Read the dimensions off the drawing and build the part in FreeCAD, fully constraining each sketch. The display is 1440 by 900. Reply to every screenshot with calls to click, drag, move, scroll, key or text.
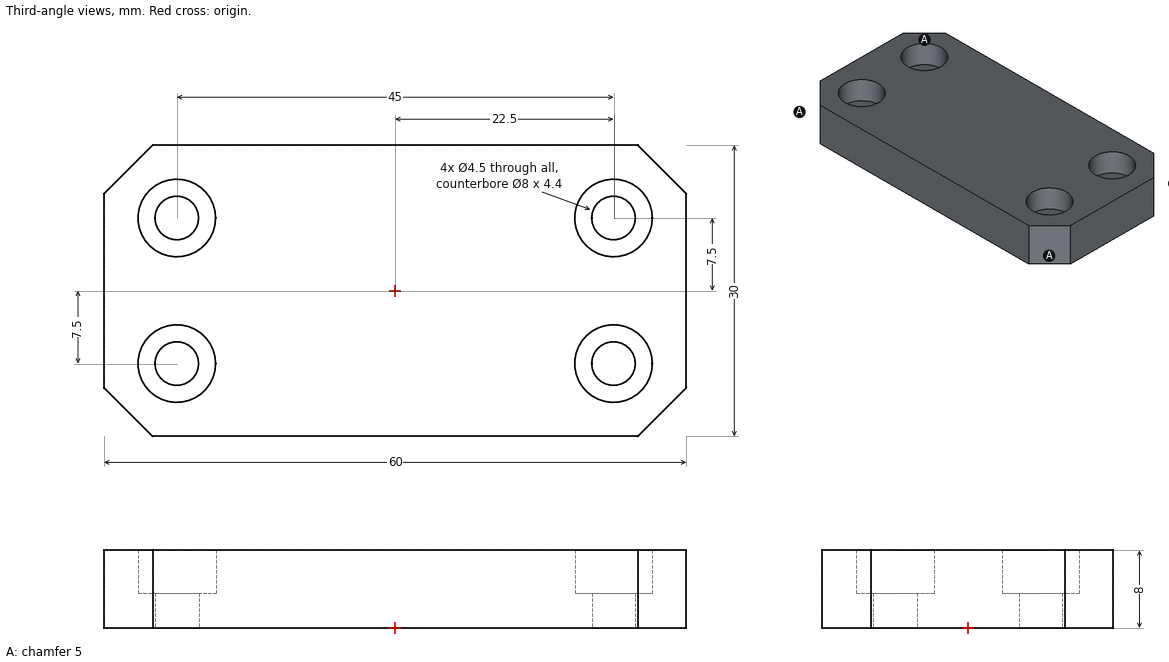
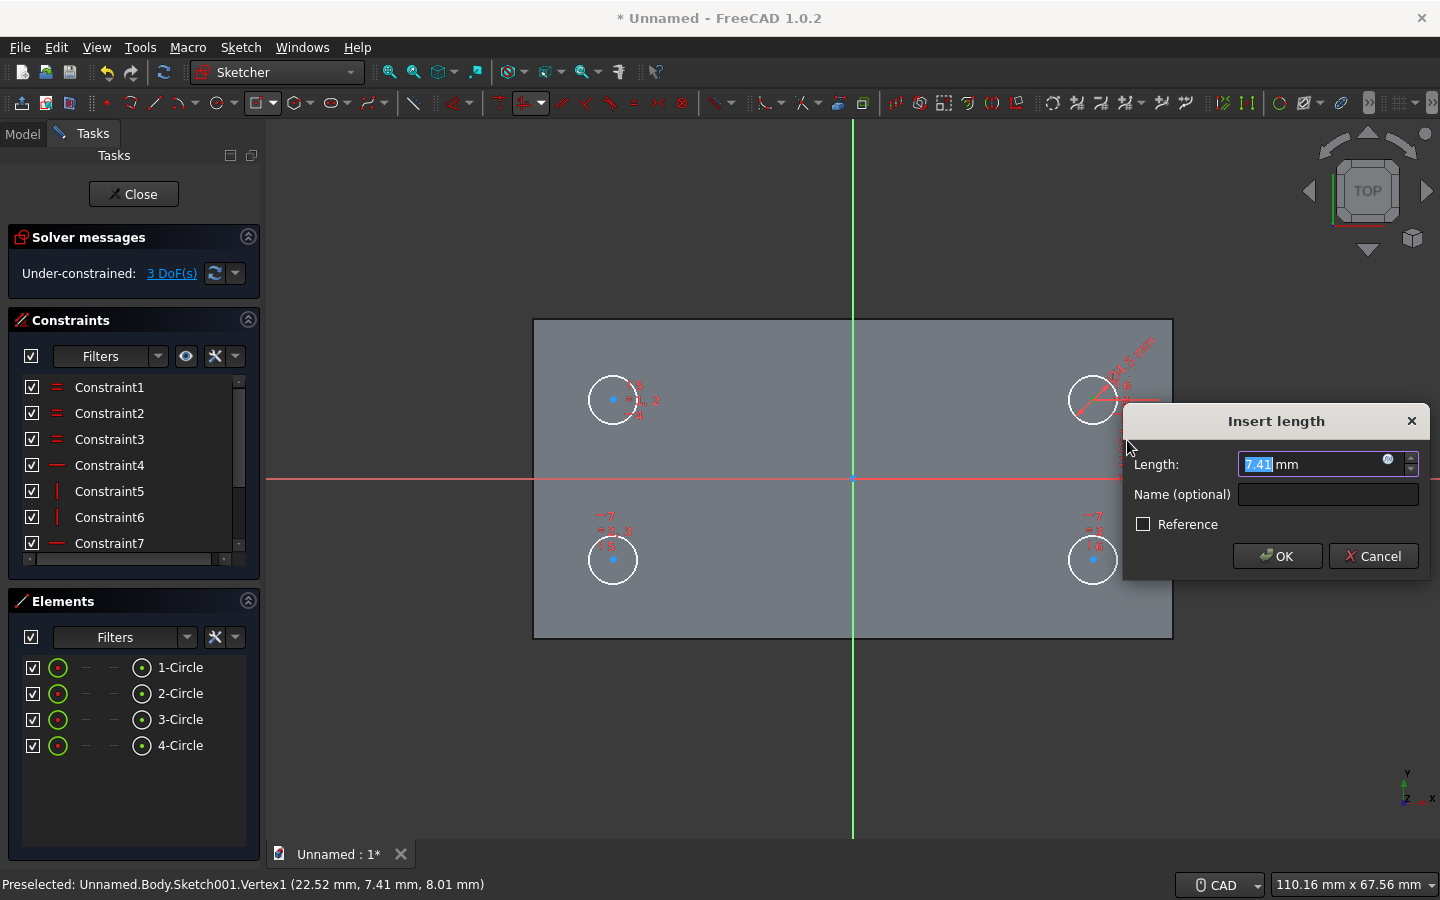
text(7.5)
key(Return)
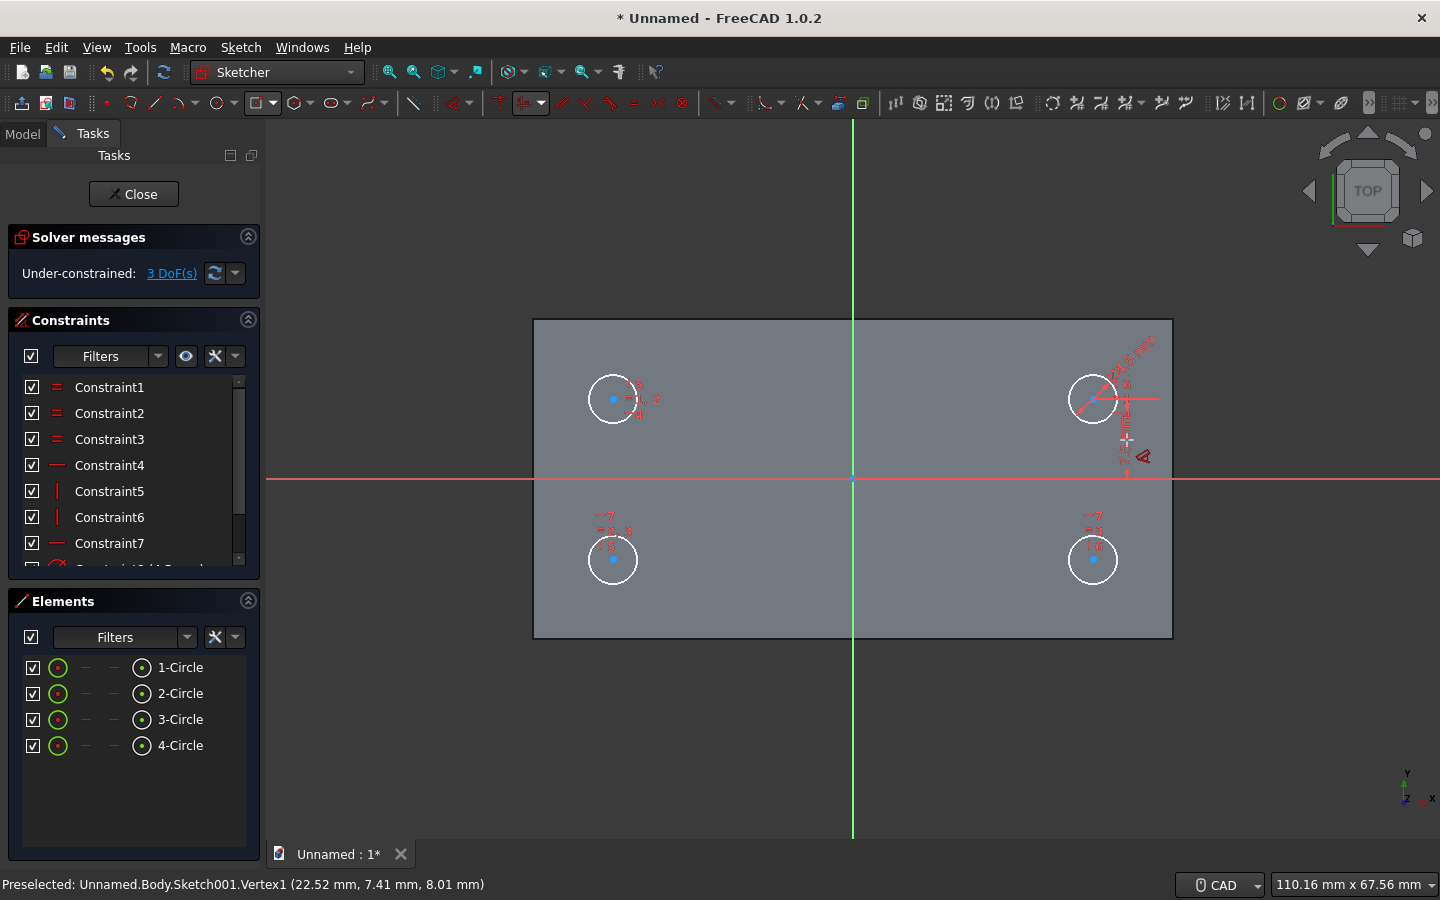
click(613, 560)
click(579, 520)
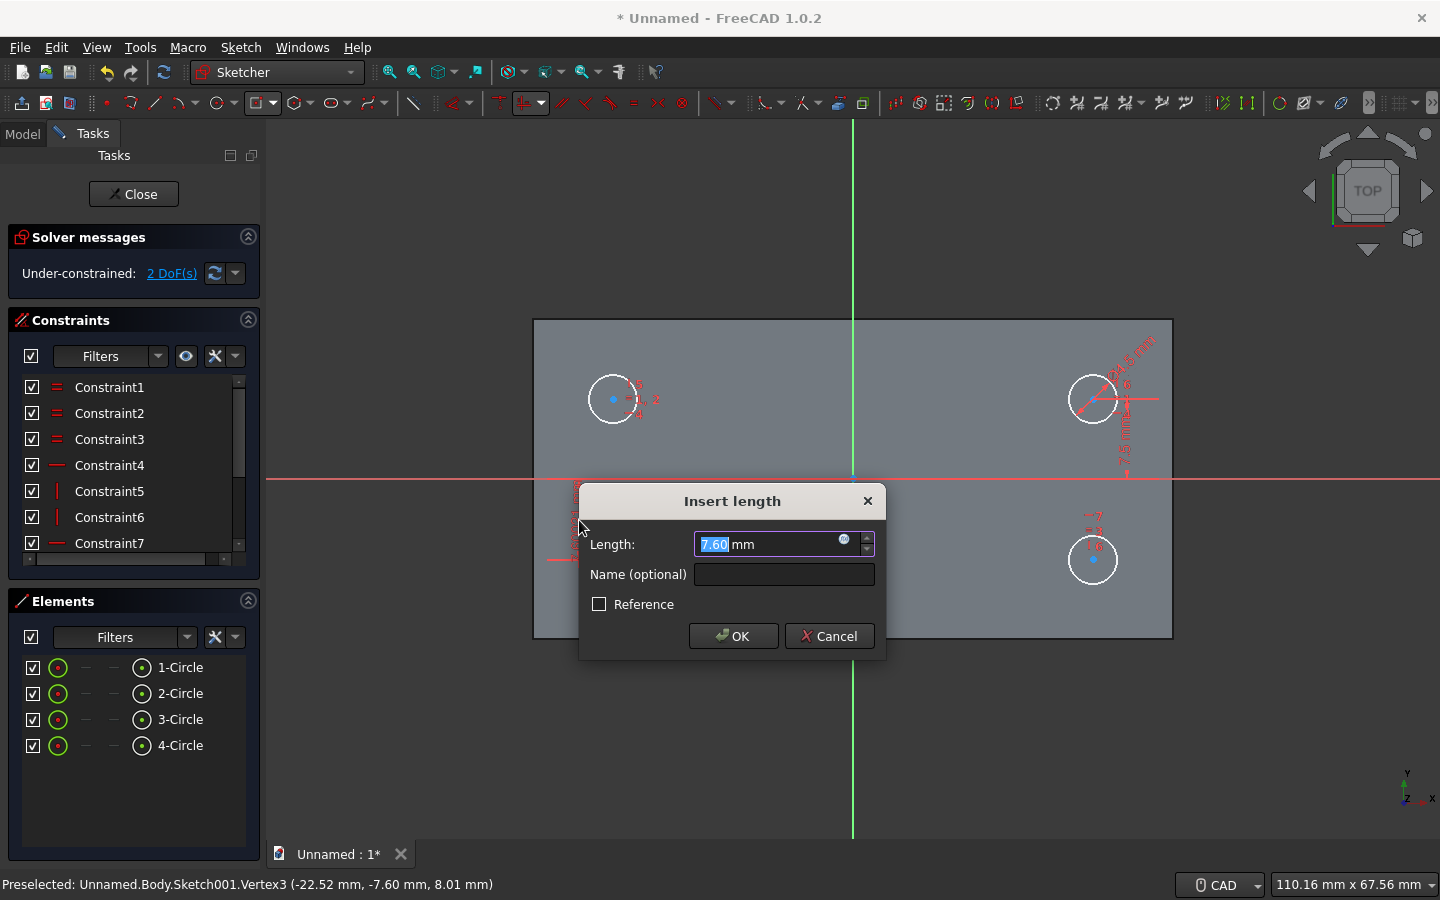
text(7.5)
key(Return)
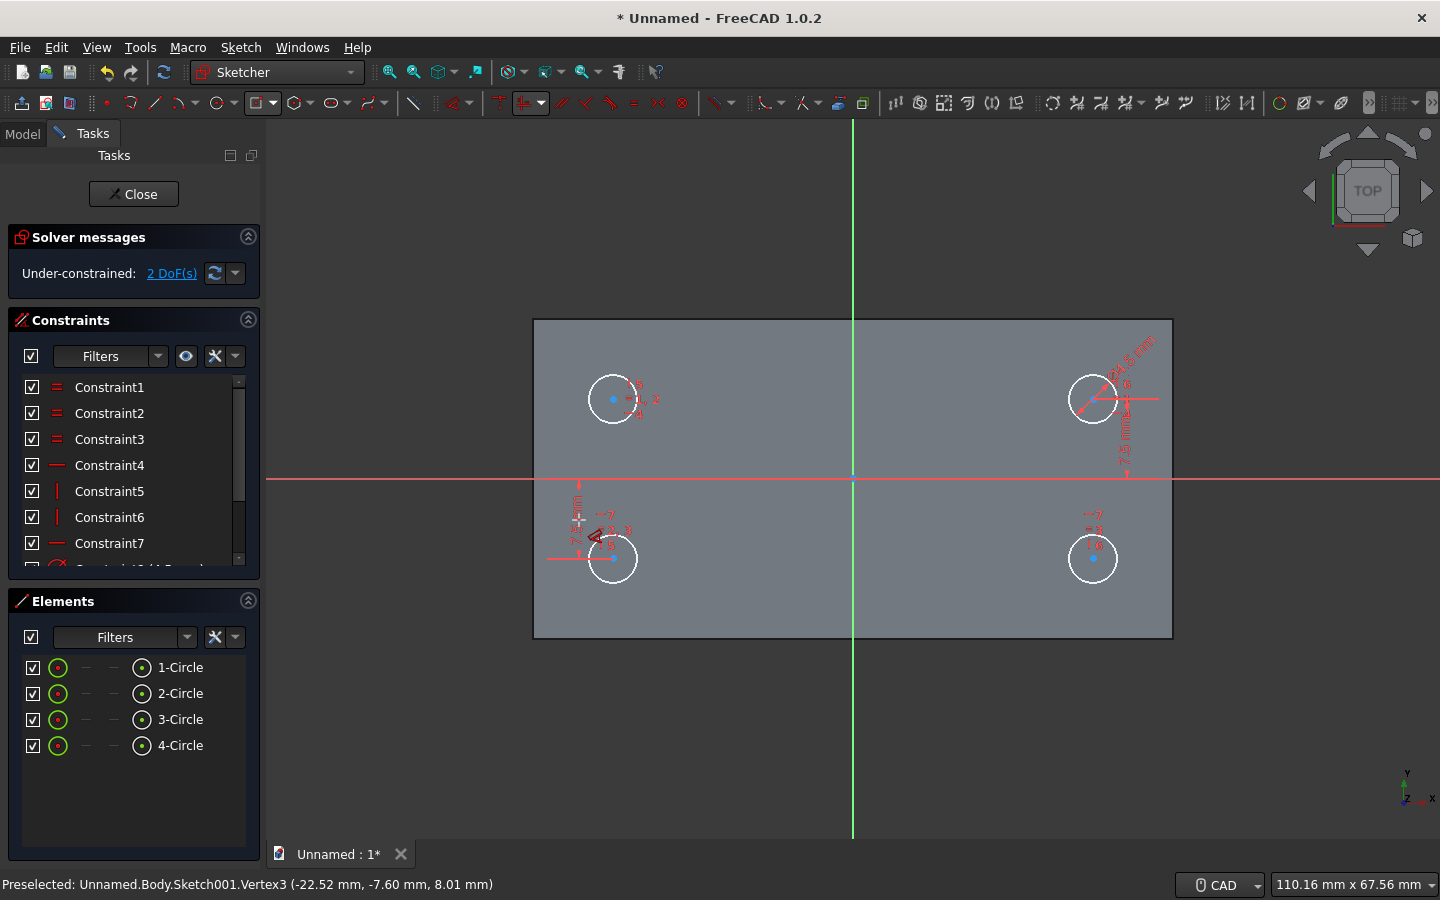
click(1093, 399)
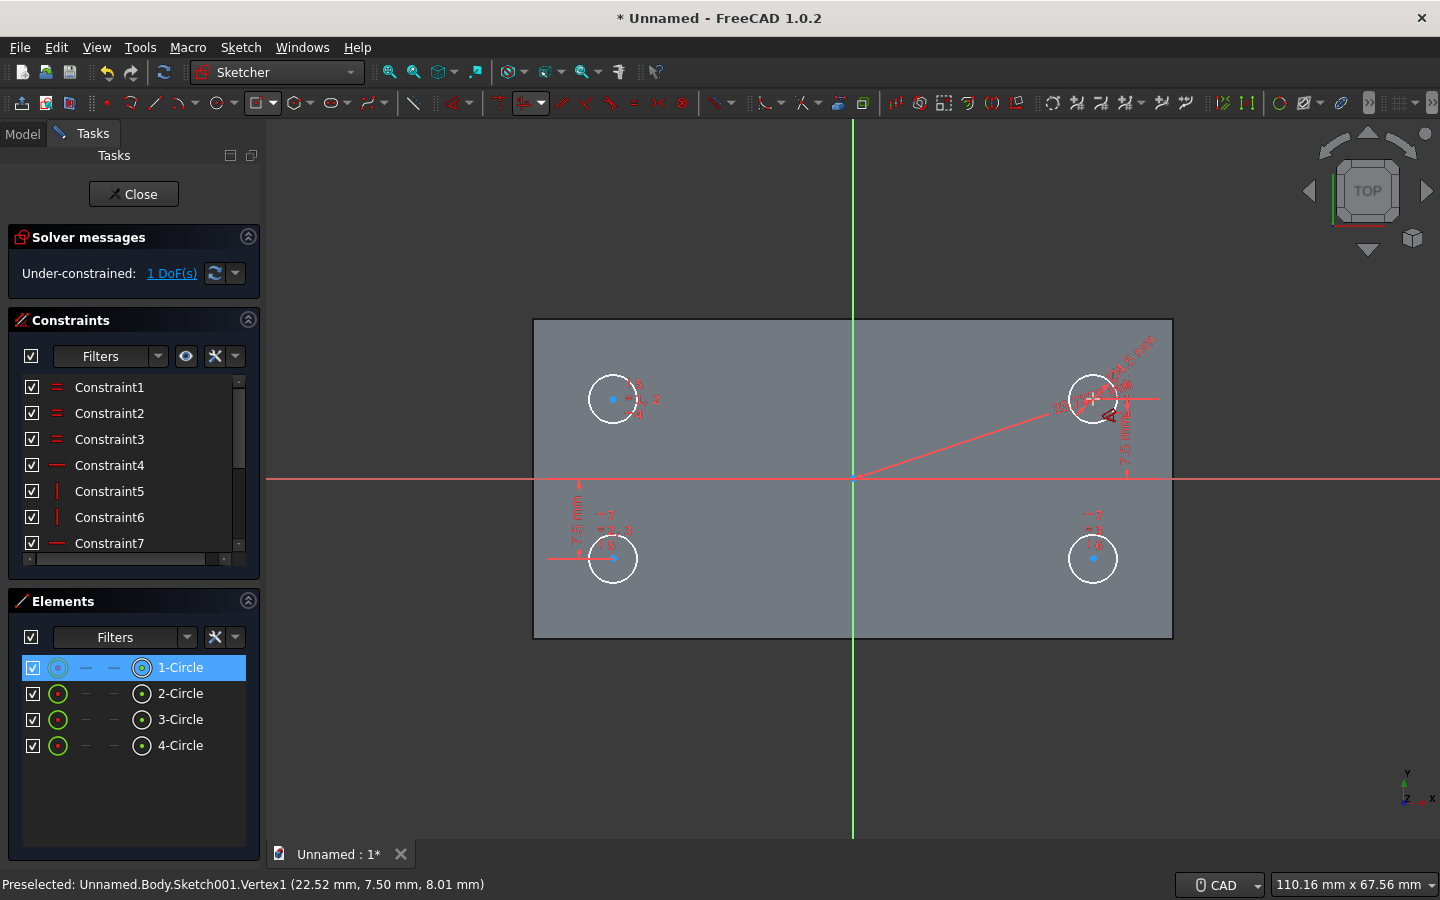
click(613, 399)
click(743, 365)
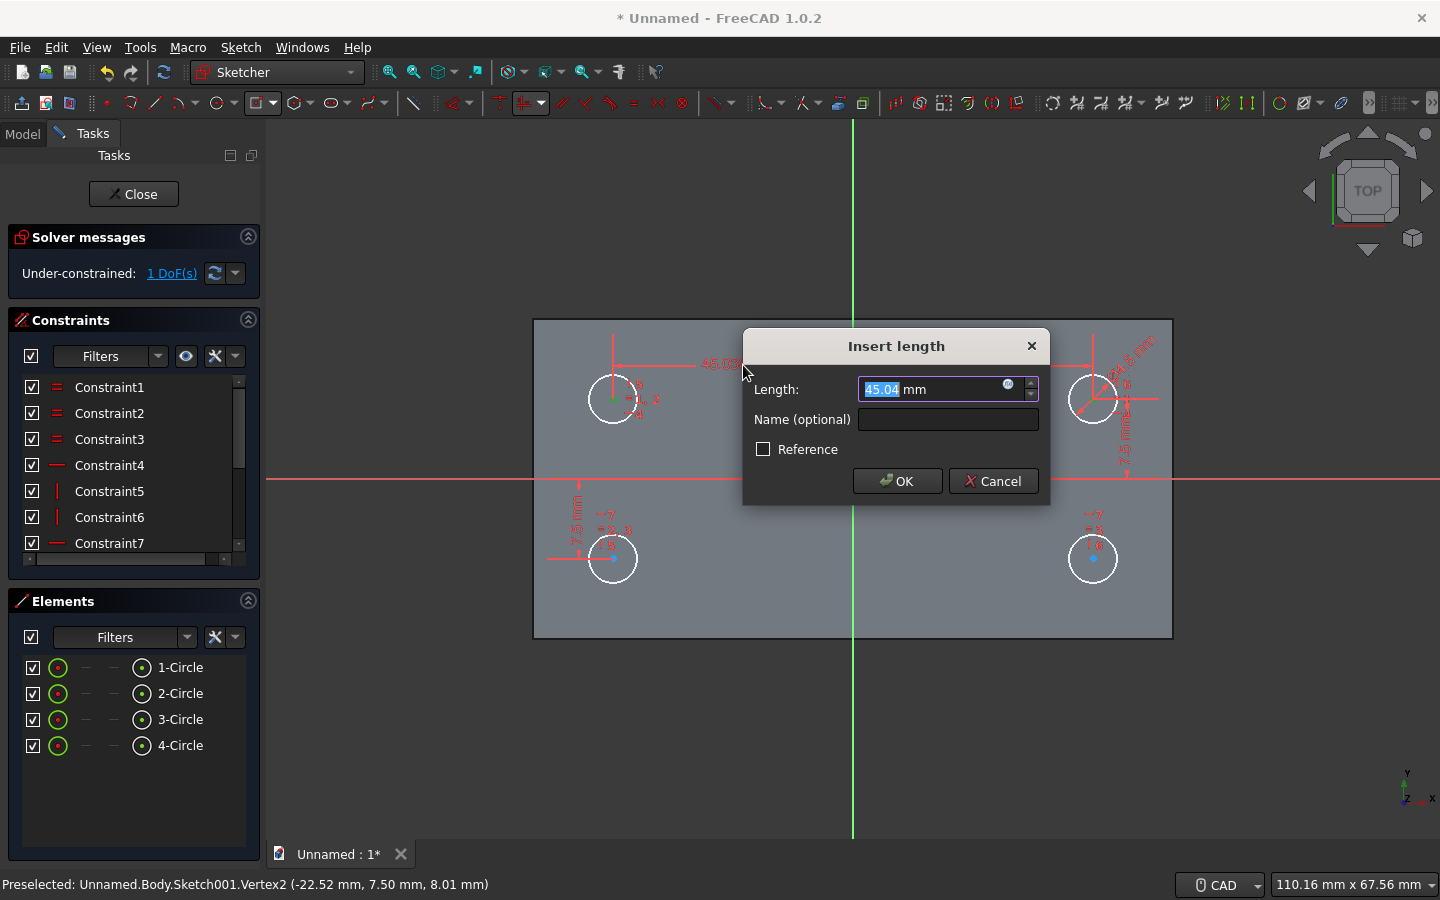
text(45)
key(Return)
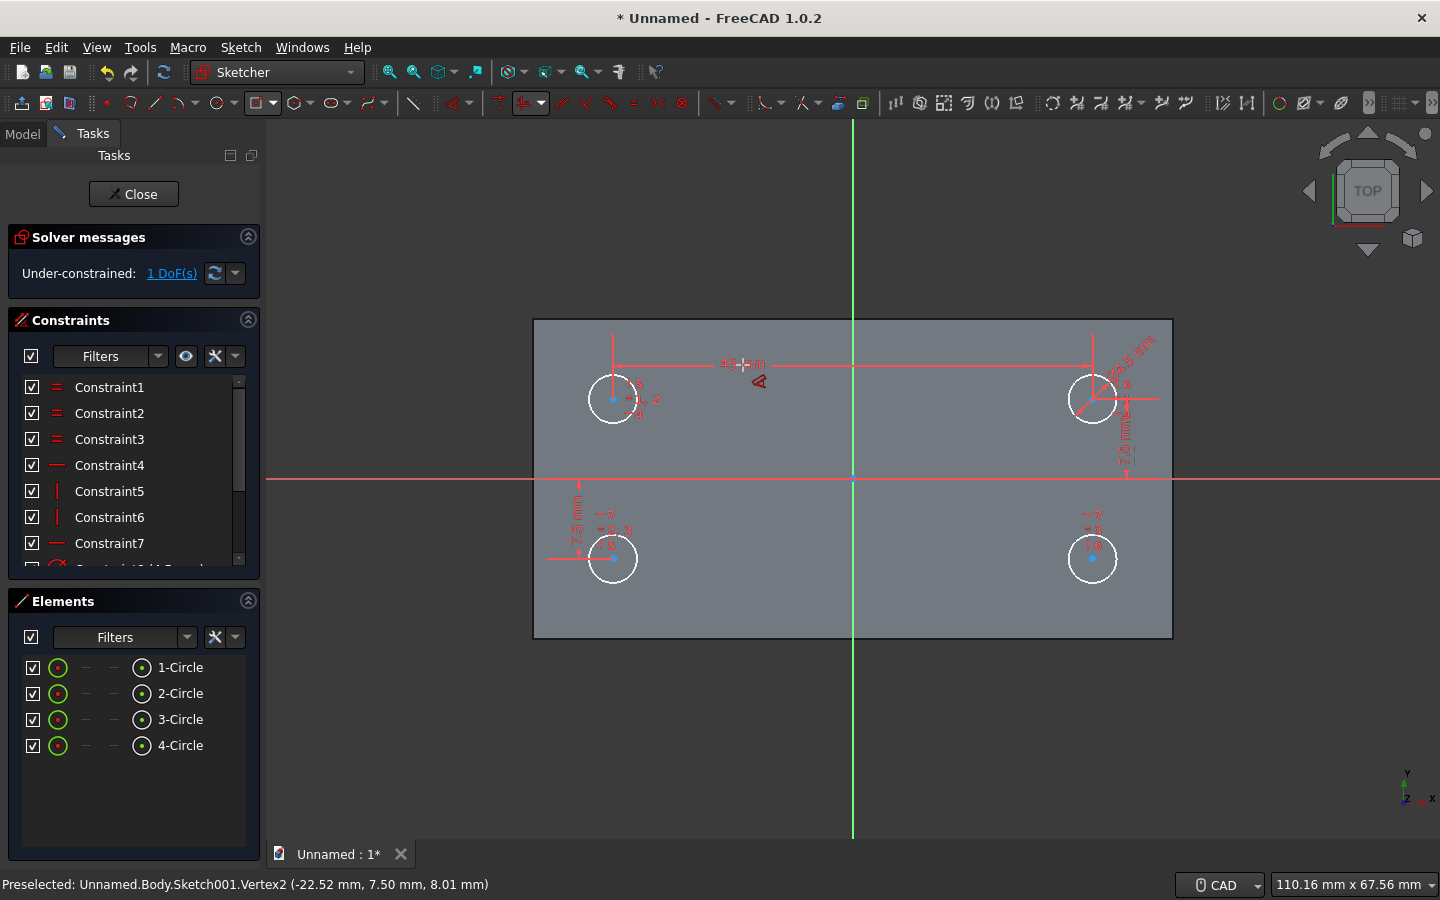
click(1093, 399)
click(973, 365)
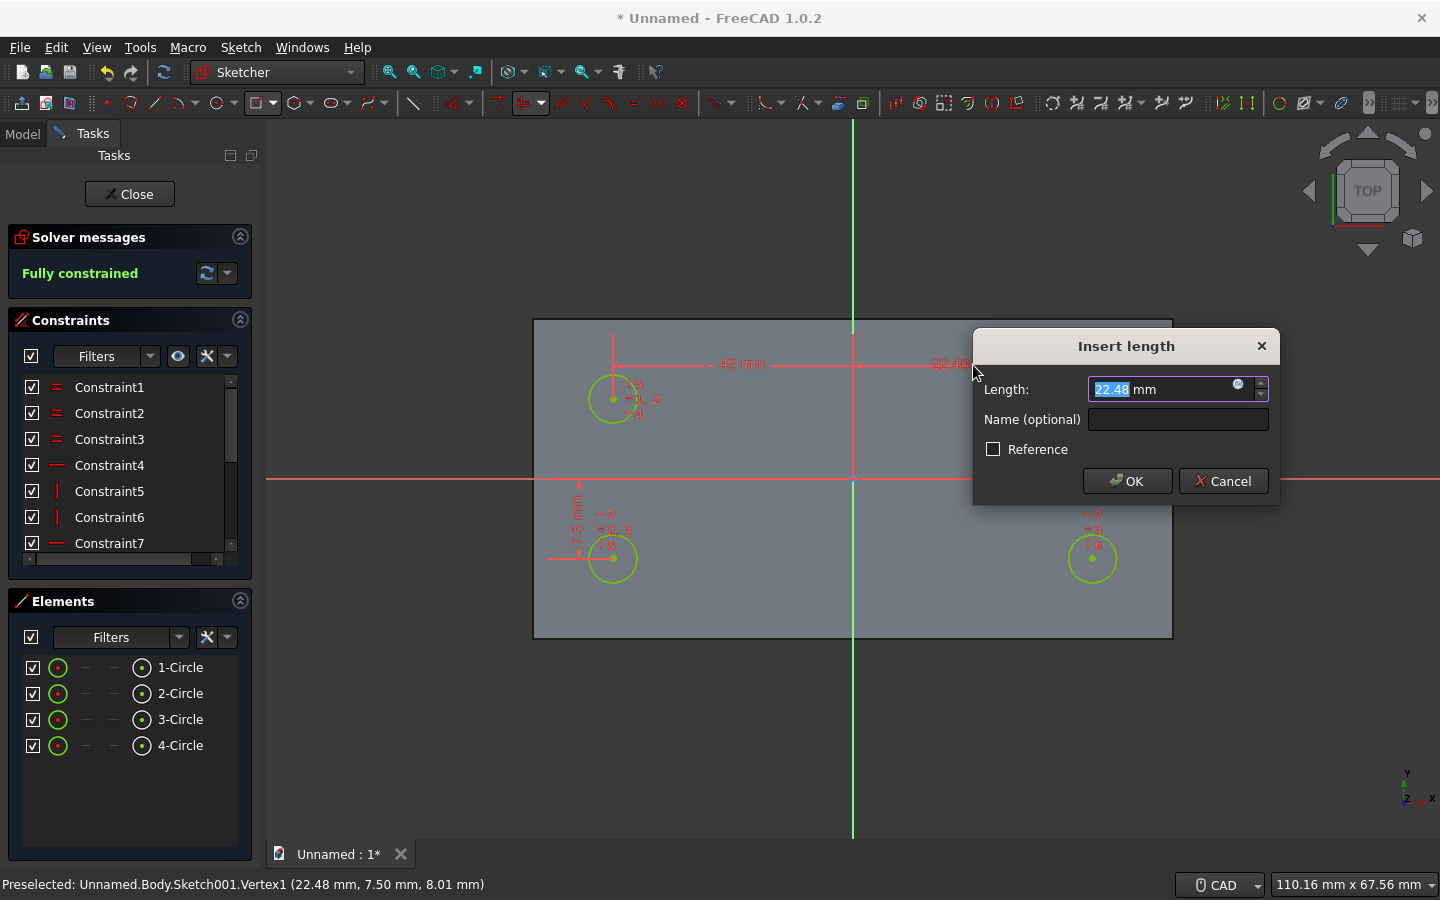
text(22.5)
key(Return)
key(Escape)